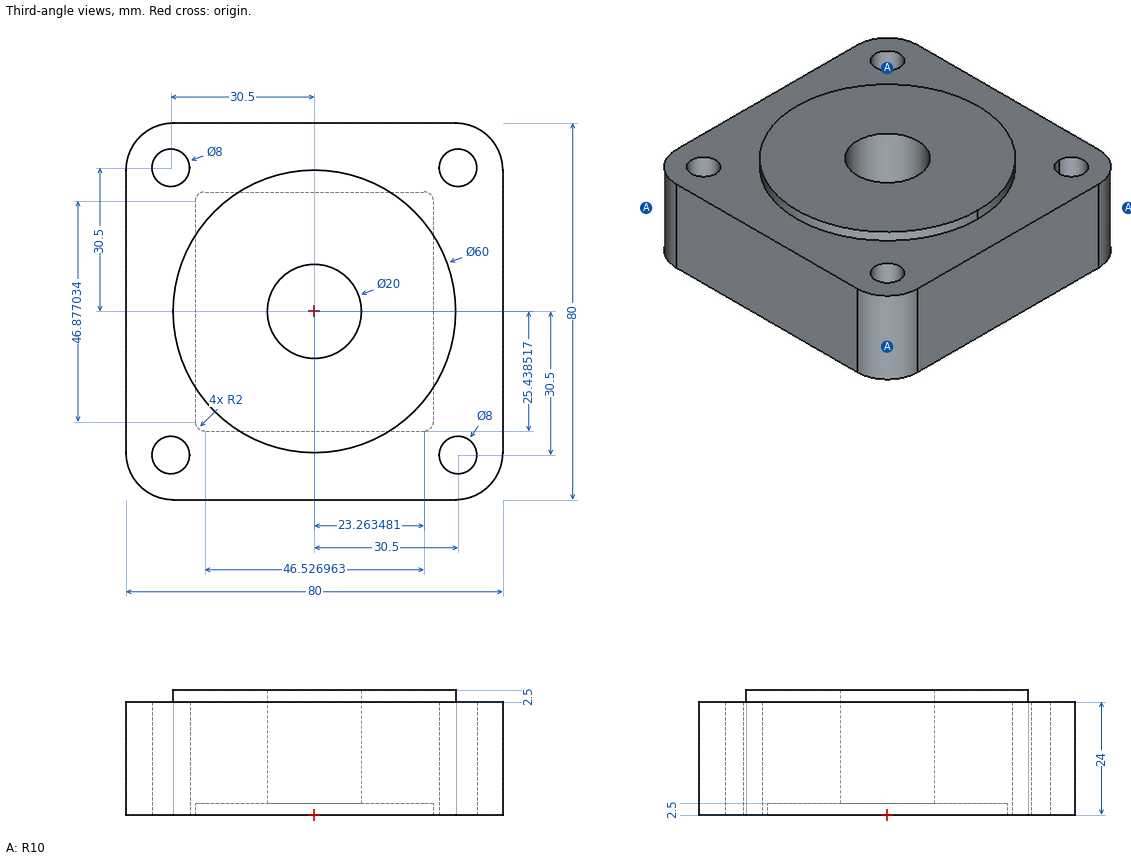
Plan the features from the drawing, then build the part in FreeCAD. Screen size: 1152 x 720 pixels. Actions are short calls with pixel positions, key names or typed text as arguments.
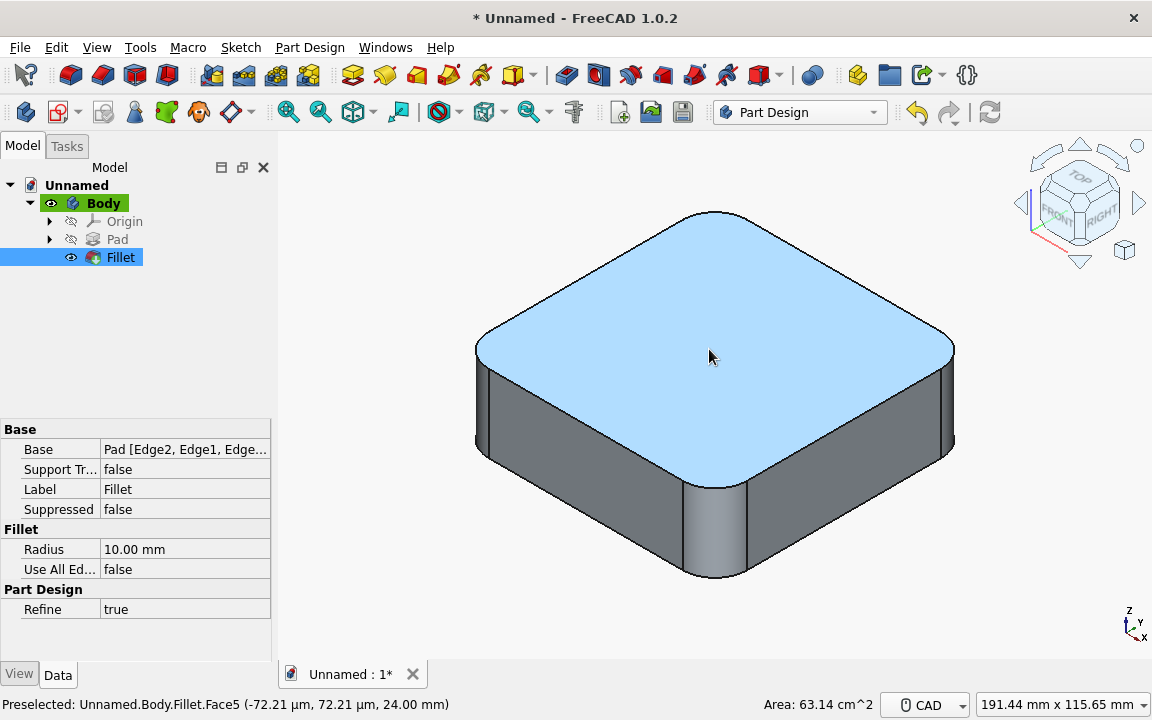
click(58, 112)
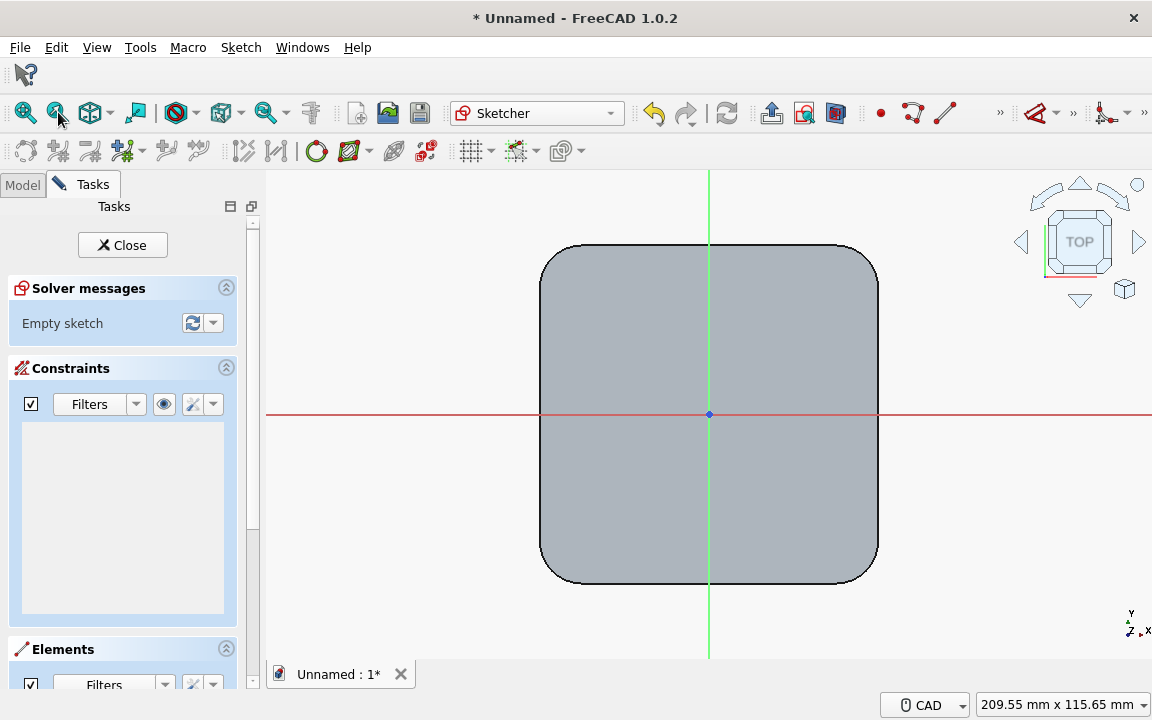
scroll(573, 269, up, 11)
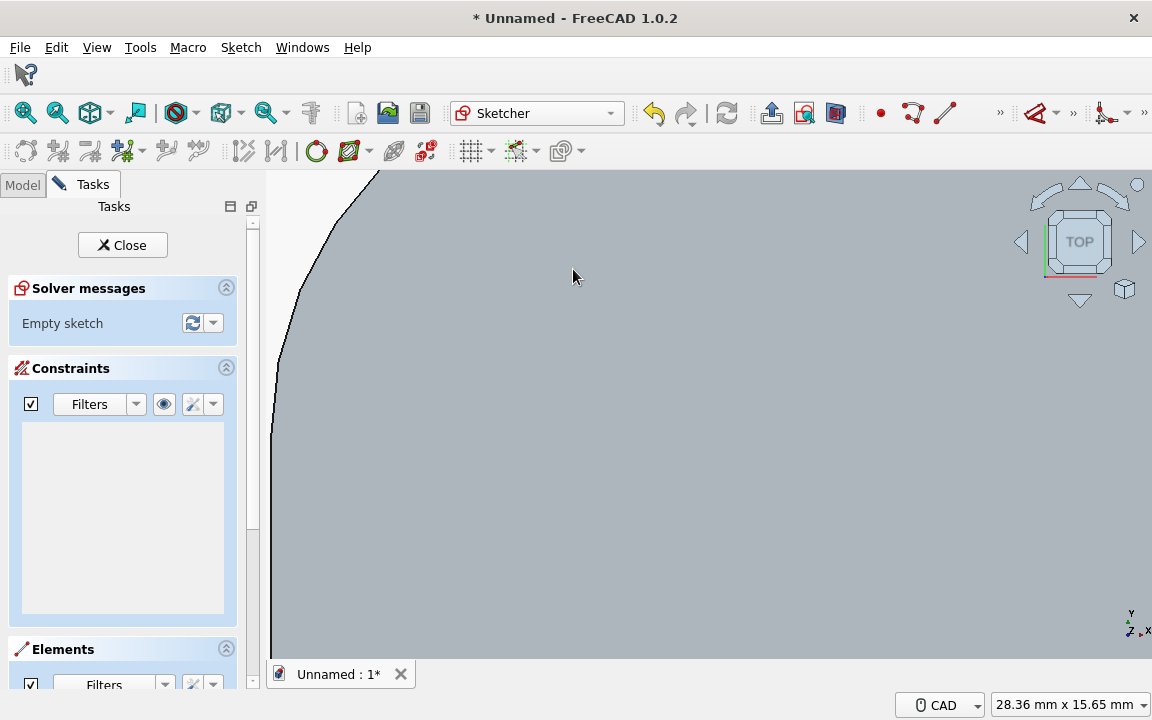
key(g)
key(c)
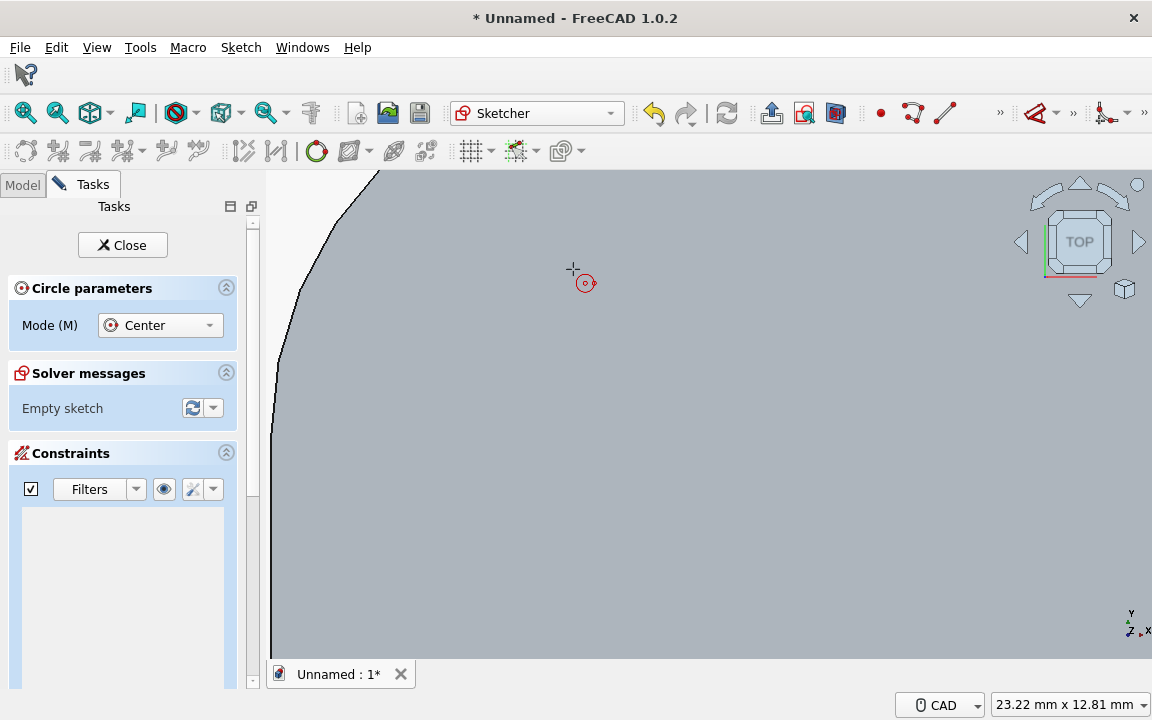
click(634, 417)
click(742, 309)
key(Escape)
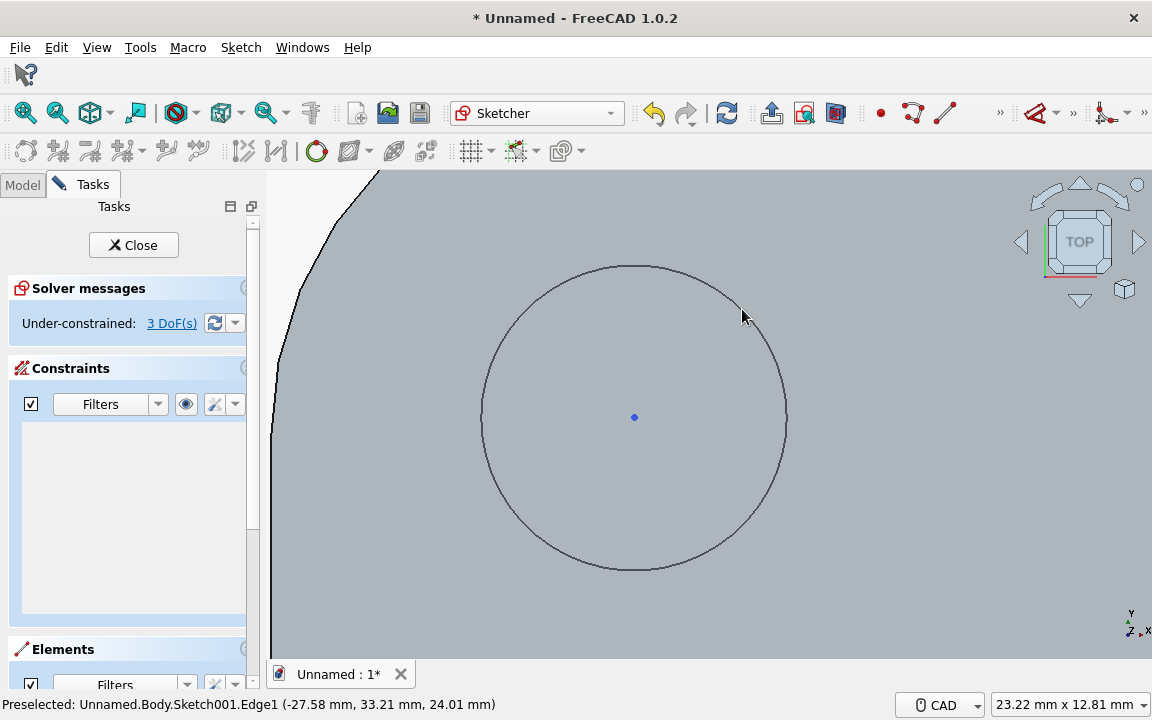
click(1036, 114)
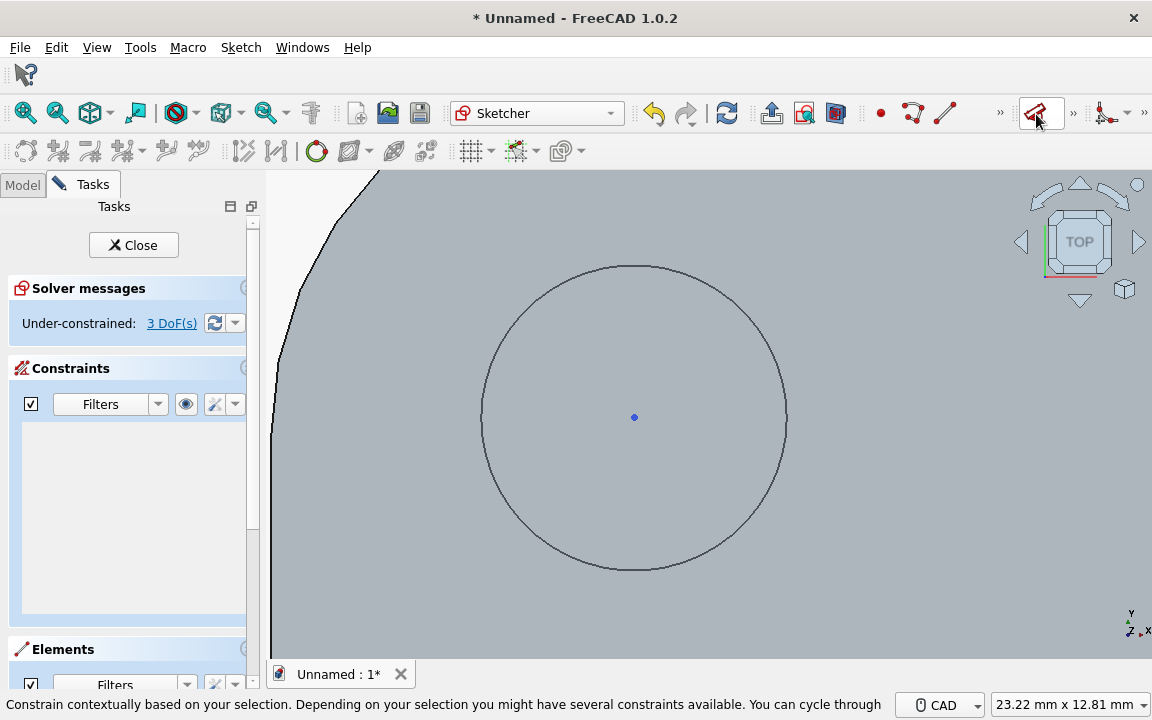
click(742, 310)
click(765, 287)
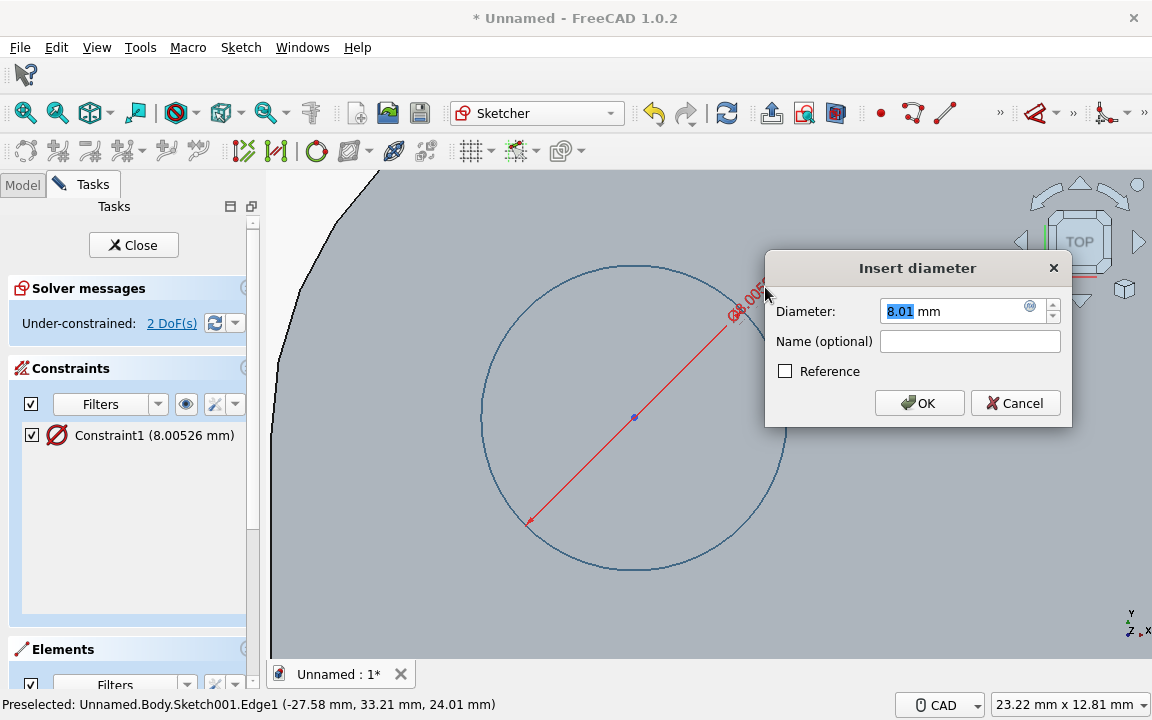
text(8)
key(Return)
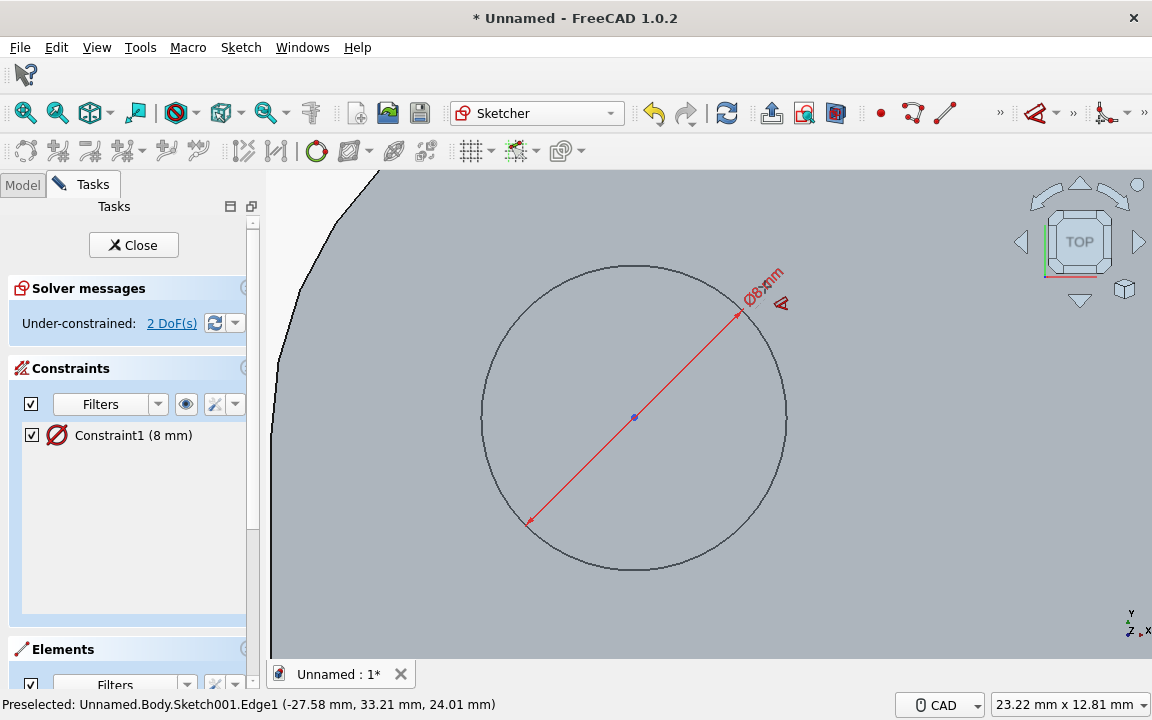
click(634, 418)
click(811, 384)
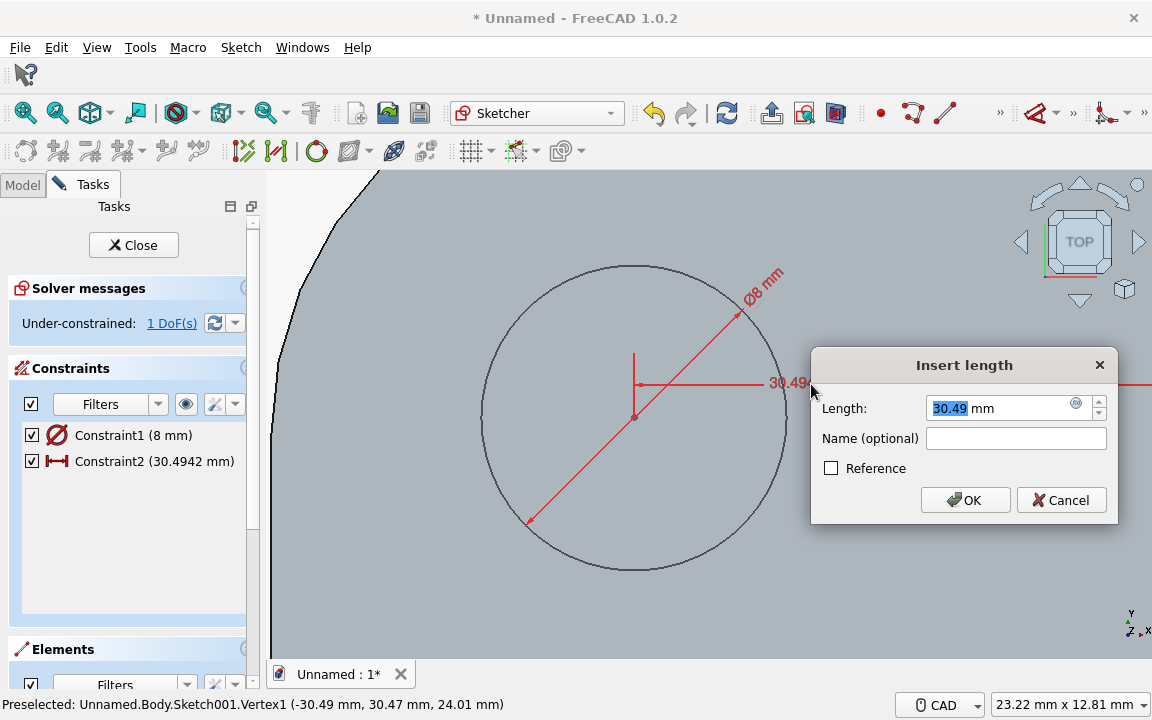
text(30.5)
key(Return)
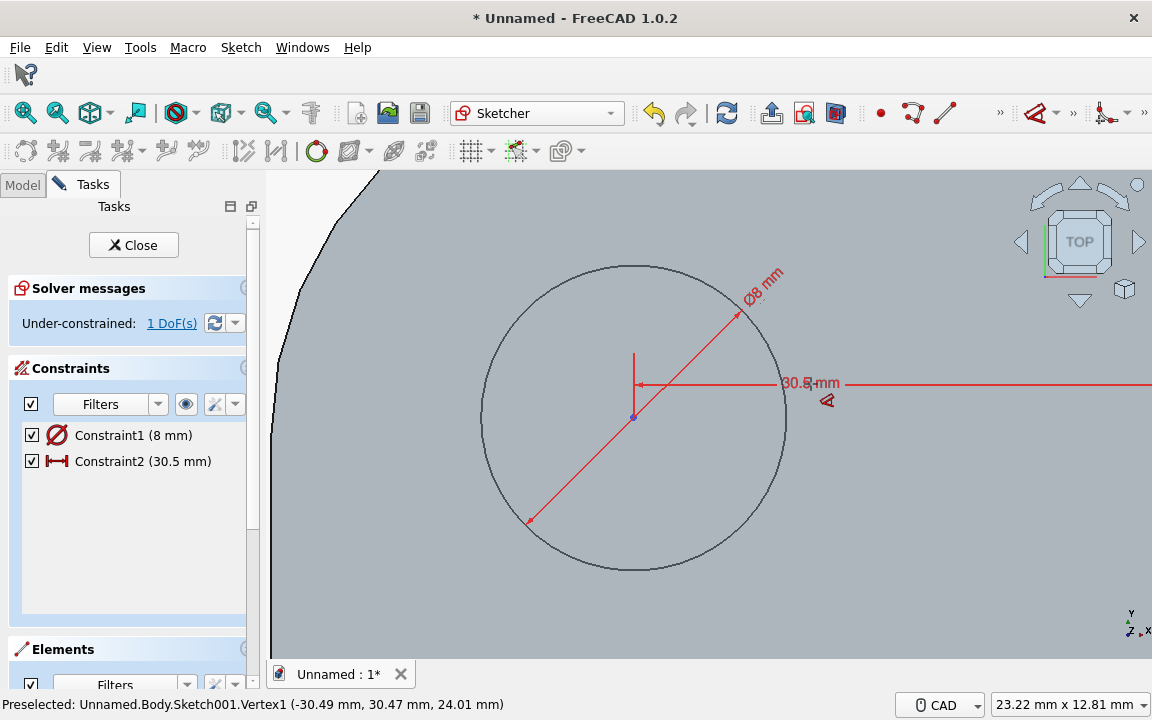
click(634, 418)
click(600, 525)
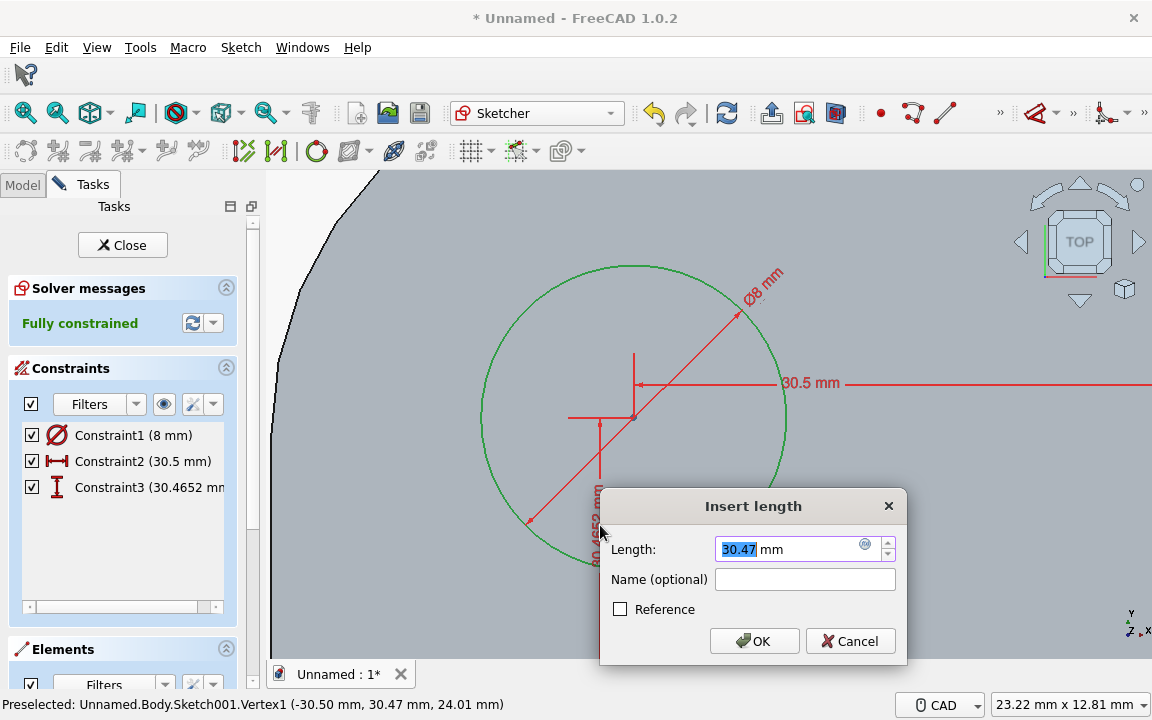
text(30.5)
key(Return)
key(Escape)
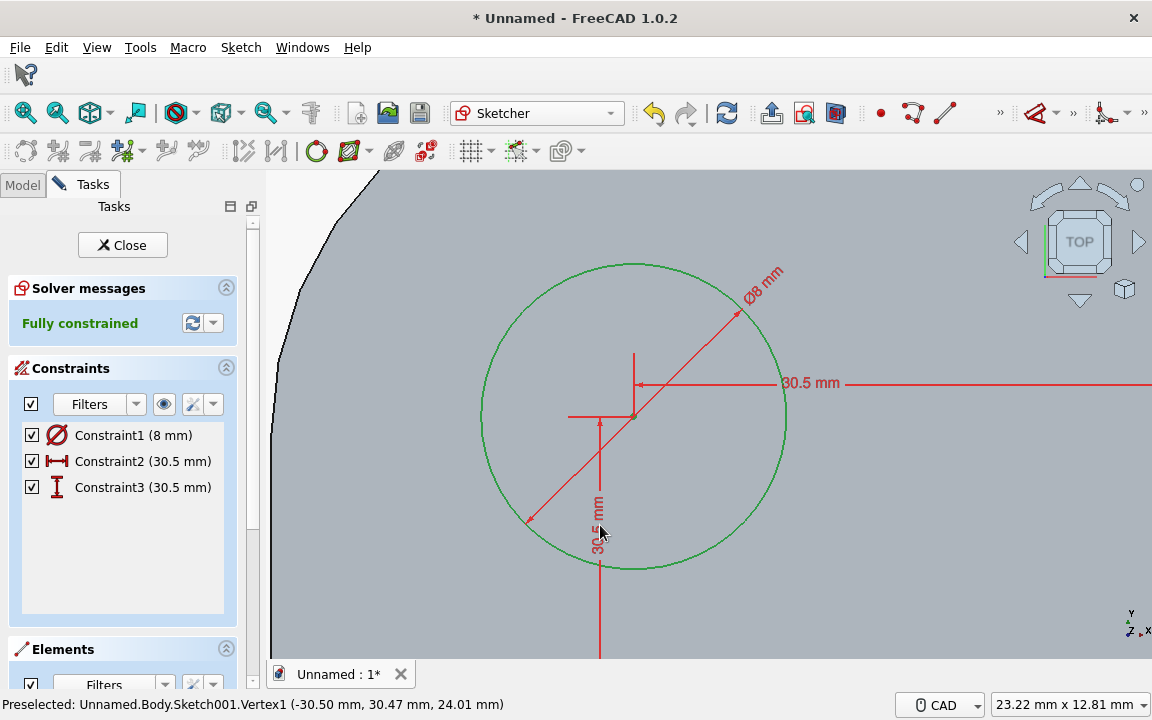
click(123, 245)